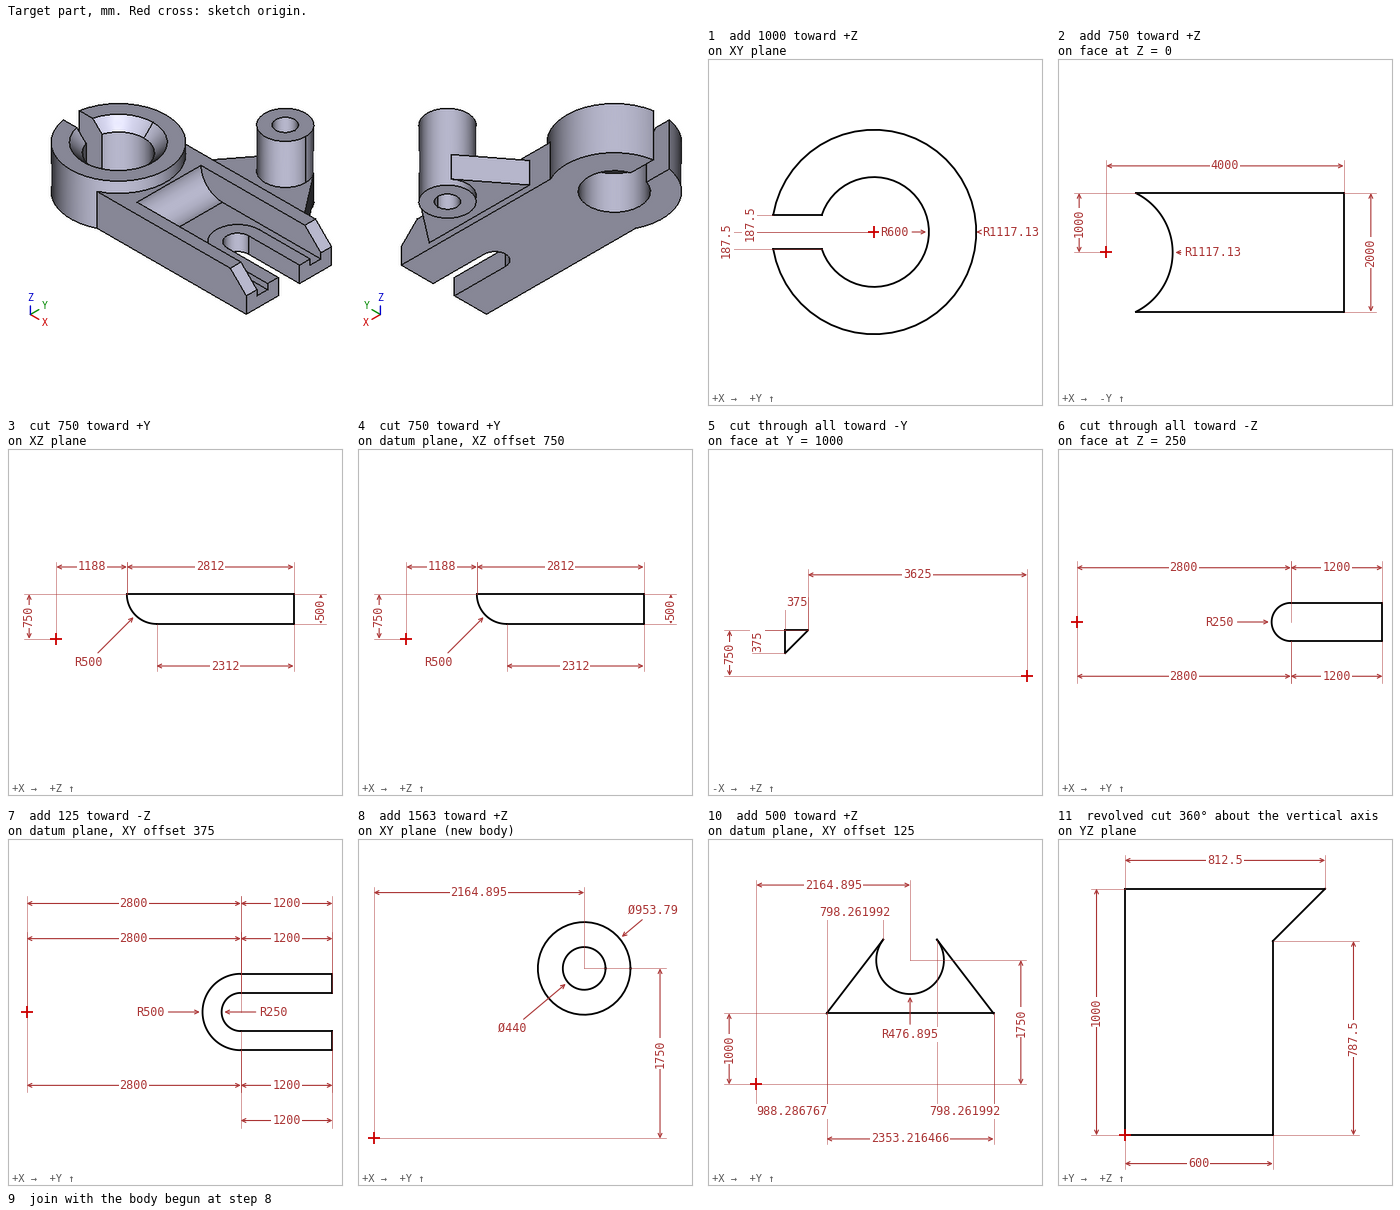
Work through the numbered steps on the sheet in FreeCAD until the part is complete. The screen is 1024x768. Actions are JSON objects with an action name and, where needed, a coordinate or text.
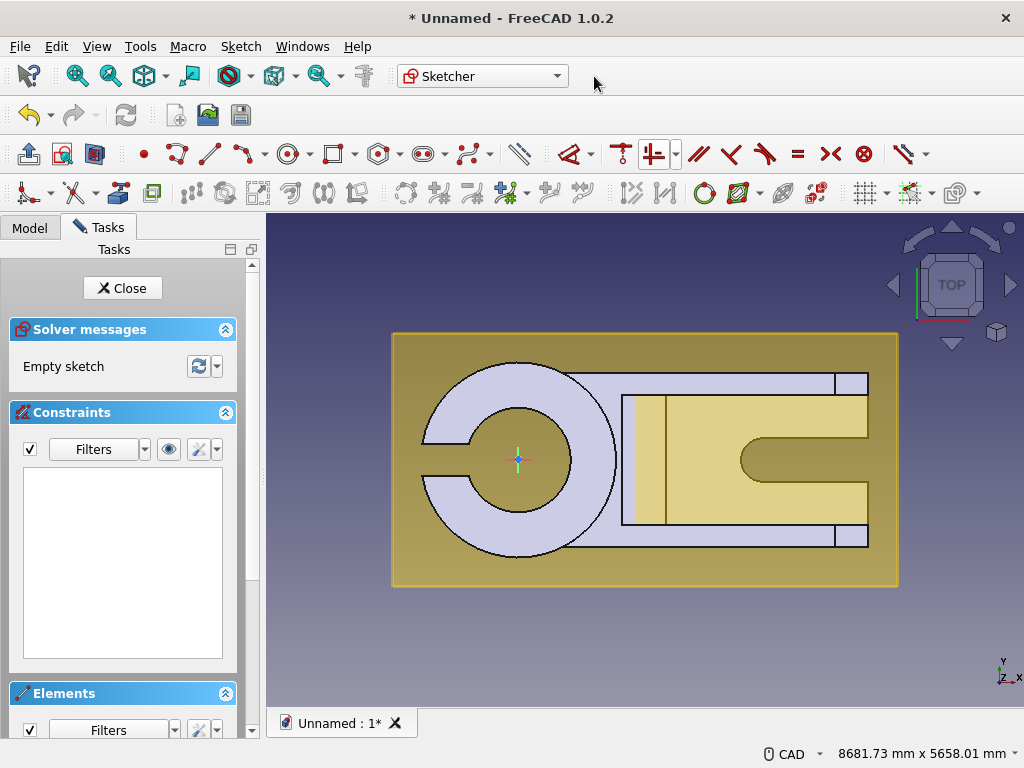
{"action": "key", "text": "q s"}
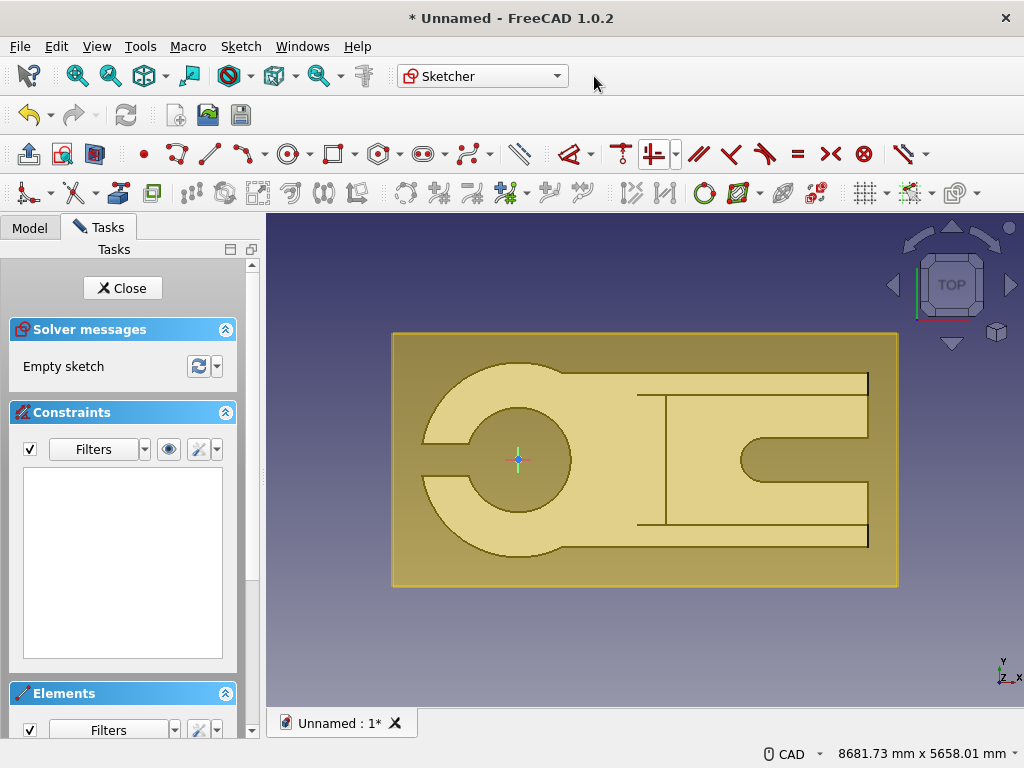
{"action": "scroll", "coordinate": [294, 460], "scroll_direction": "down", "scroll_amount": 1}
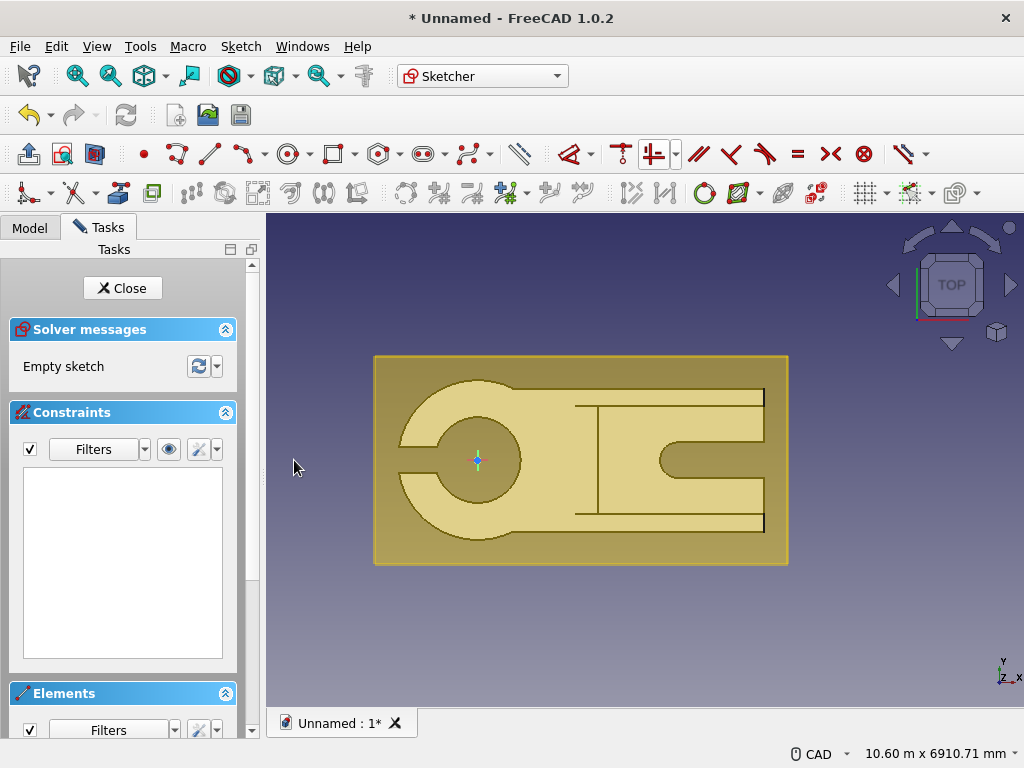
{"action": "scroll", "coordinate": [711, 460], "scroll_direction": "up", "scroll_amount": 2}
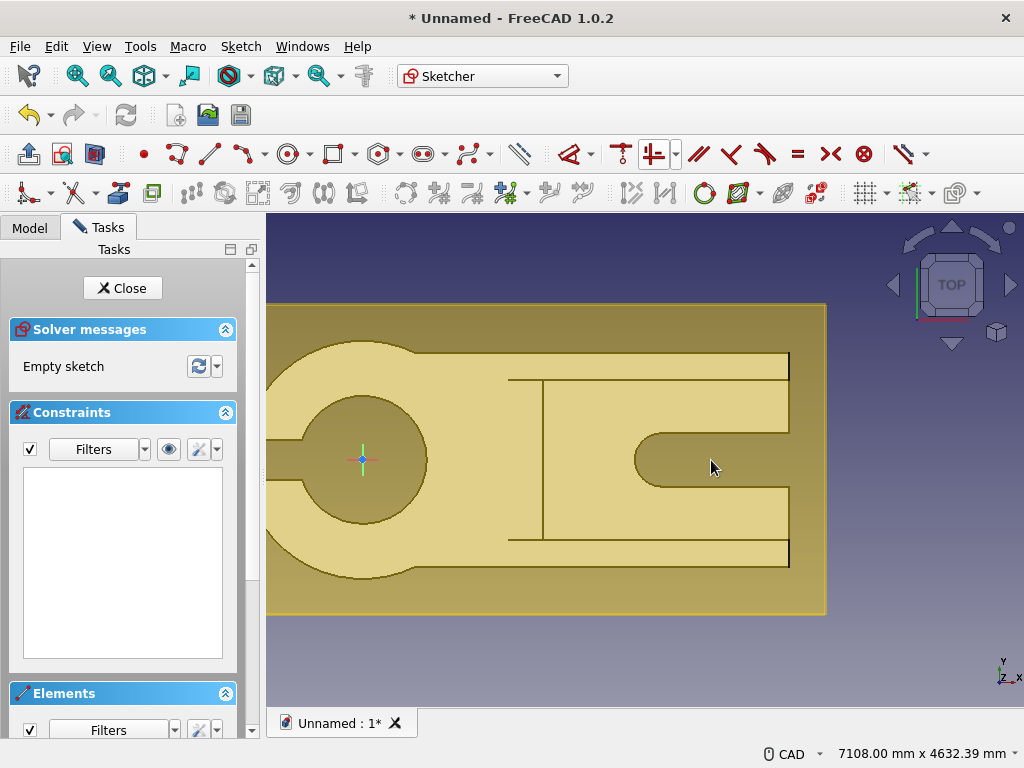
{"action": "left_click", "coordinate": [177, 154]}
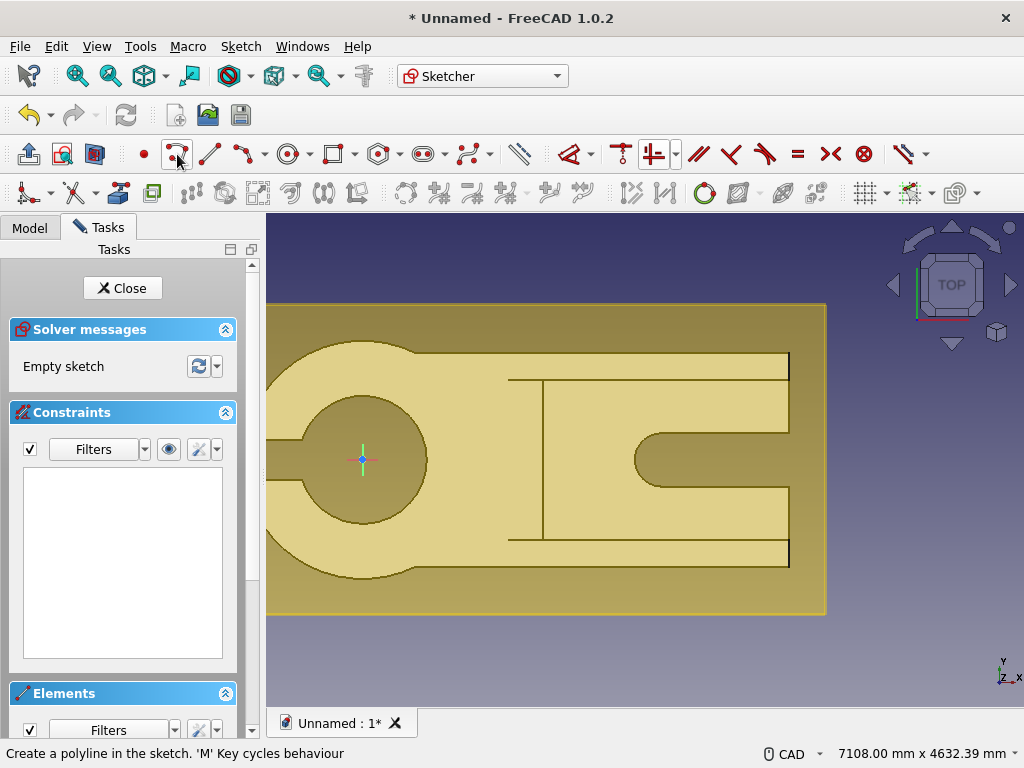
{"action": "left_click", "coordinate": [661, 433]}
{"action": "left_click", "coordinate": [789, 433]}
{"action": "left_click", "coordinate": [789, 407]}
{"action": "left_click", "coordinate": [661, 407]}
{"action": "right_click", "coordinate": [661, 407]}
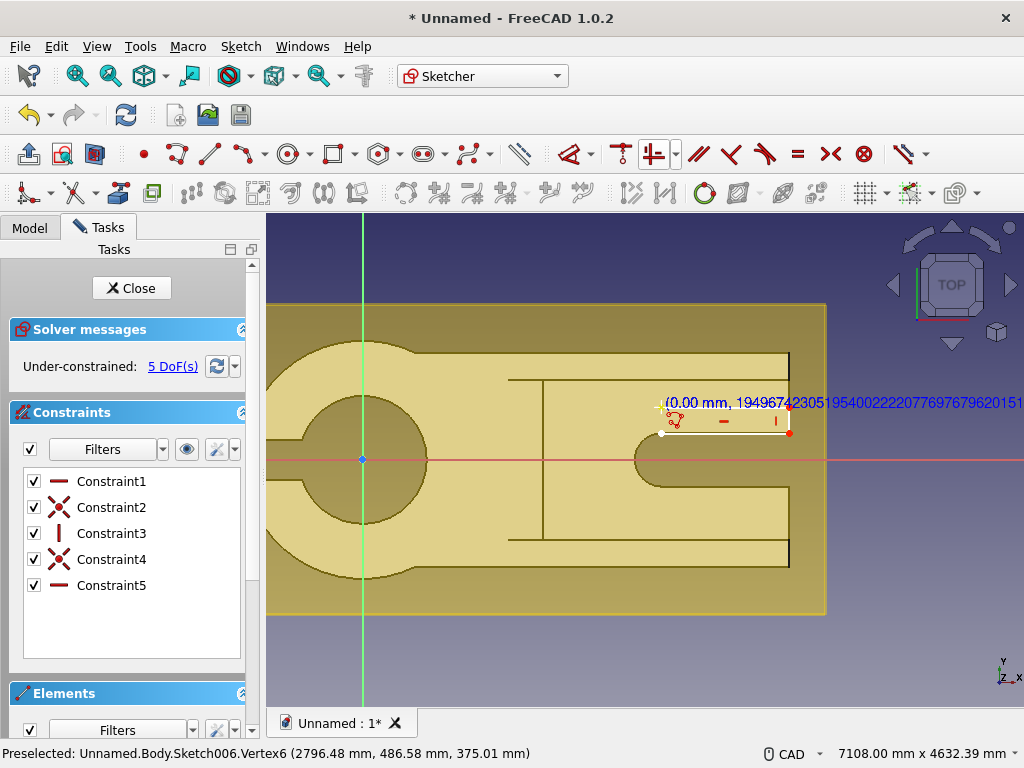
{"action": "left_click", "coordinate": [661, 513]}
{"action": "left_click", "coordinate": [789, 513]}
{"action": "left_click", "coordinate": [789, 487]}
{"action": "left_click", "coordinate": [661, 487]}
{"action": "right_click", "coordinate": [661, 487]}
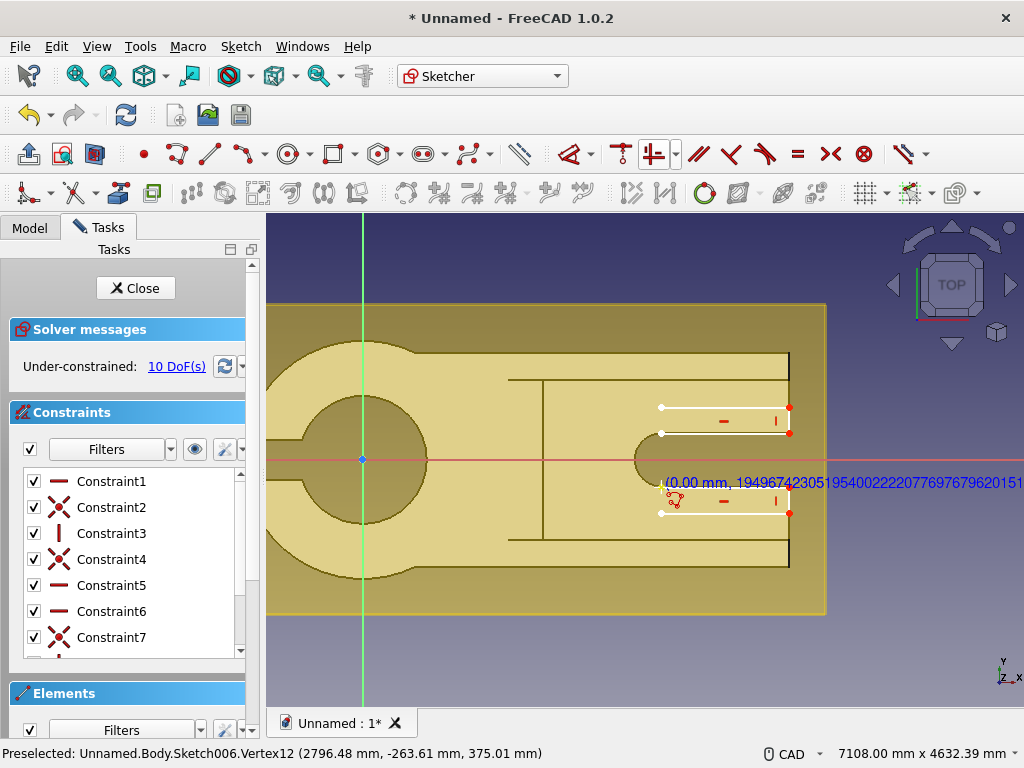
{"action": "key", "text": "g 3 a"}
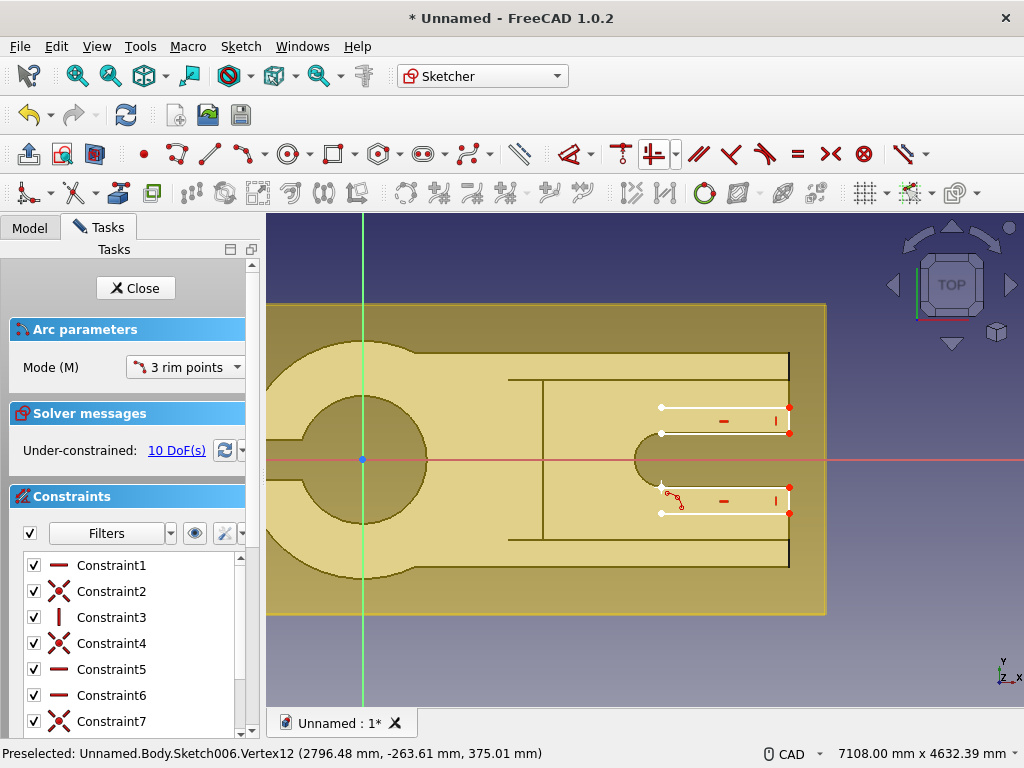
{"action": "left_click", "coordinate": [661, 408]}
{"action": "left_click", "coordinate": [661, 514]}
{"action": "left_click", "coordinate": [611, 443]}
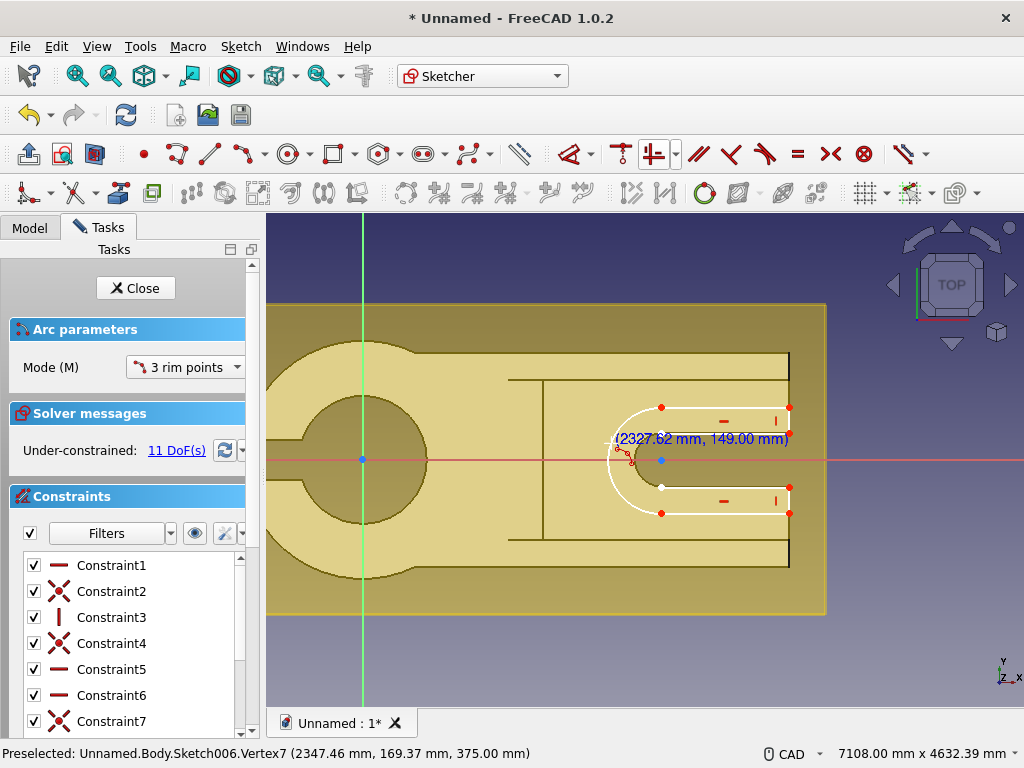
{"action": "left_click", "coordinate": [661, 488]}
{"action": "left_click", "coordinate": [661, 434]}
{"action": "left_click", "coordinate": [640, 444]}
{"action": "key", "text": "Escape"}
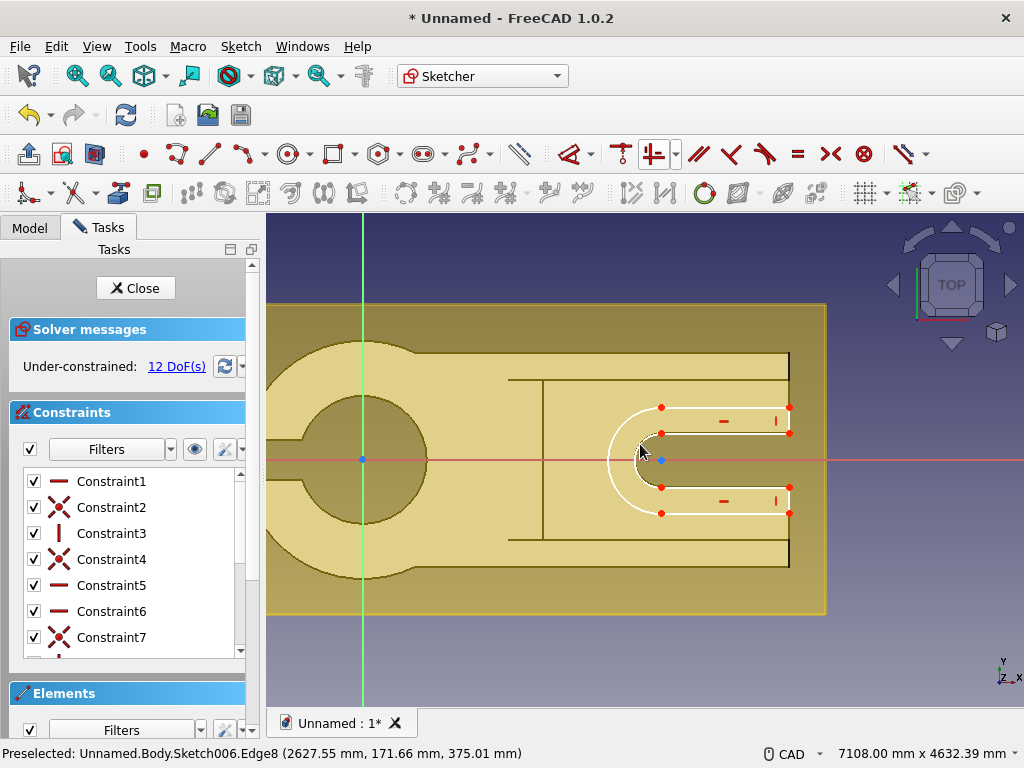
{"action": "left_click", "coordinate": [618, 430]}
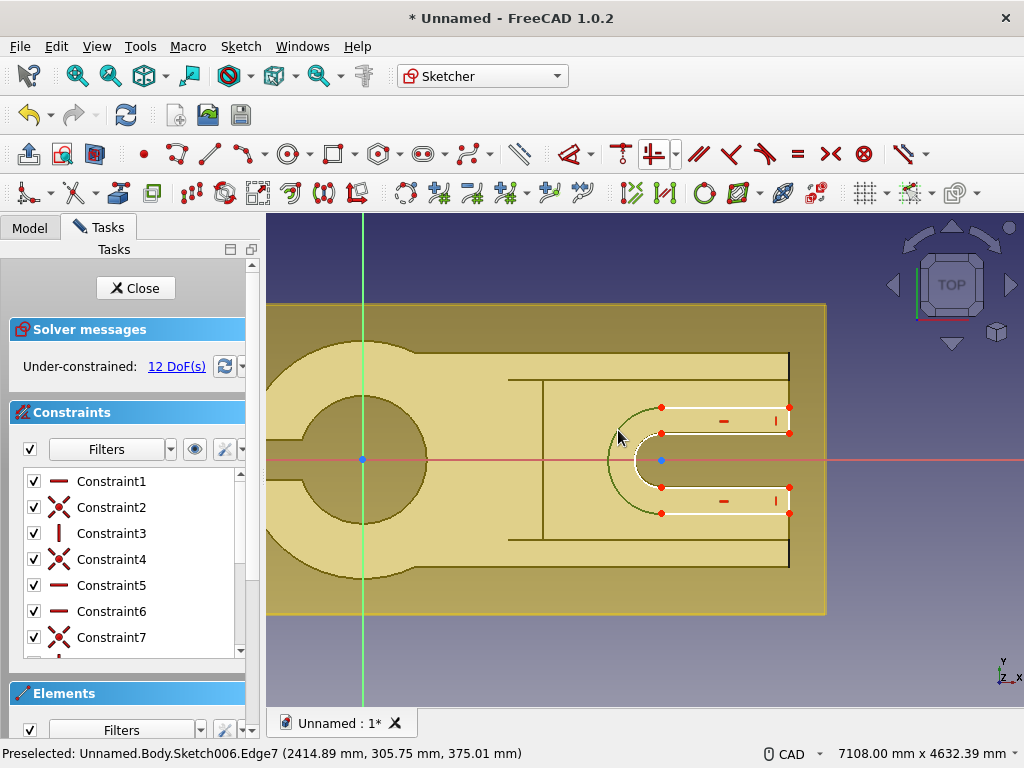
{"action": "left_click", "coordinate": [640, 445]}